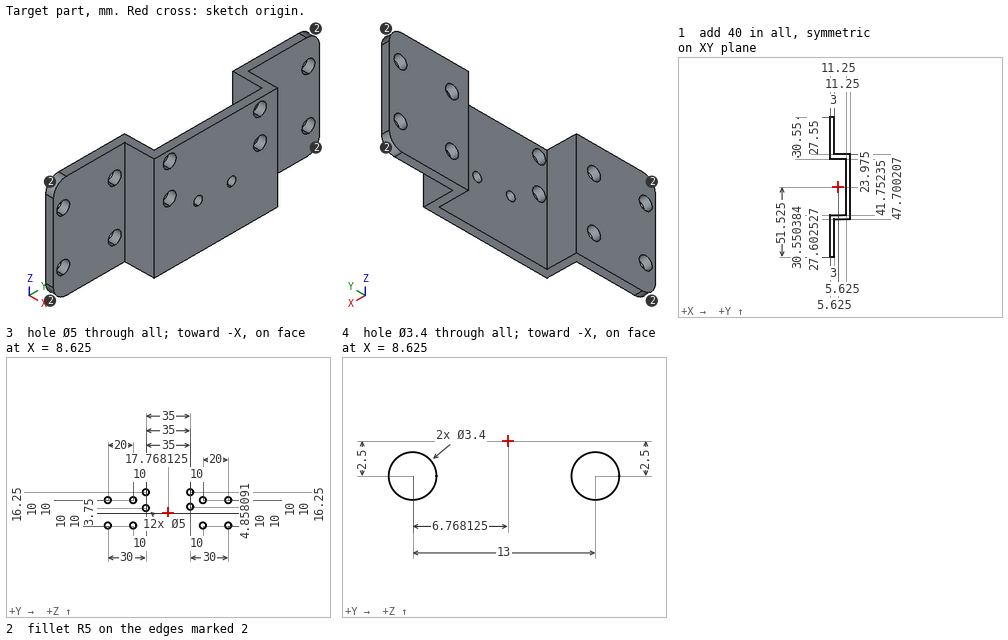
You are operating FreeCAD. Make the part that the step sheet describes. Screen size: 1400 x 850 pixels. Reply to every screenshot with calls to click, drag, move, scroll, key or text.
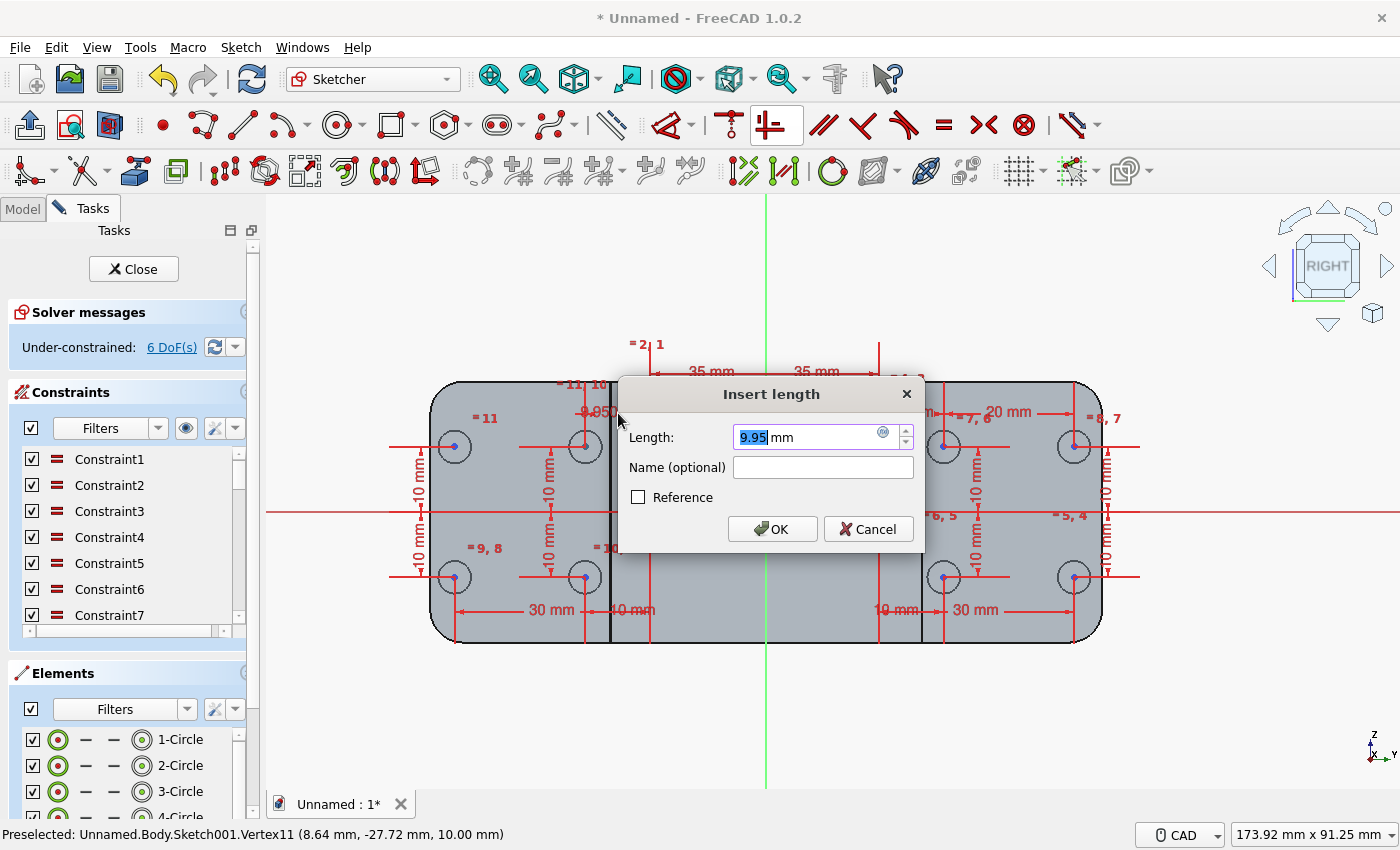
text(10)
key(Return)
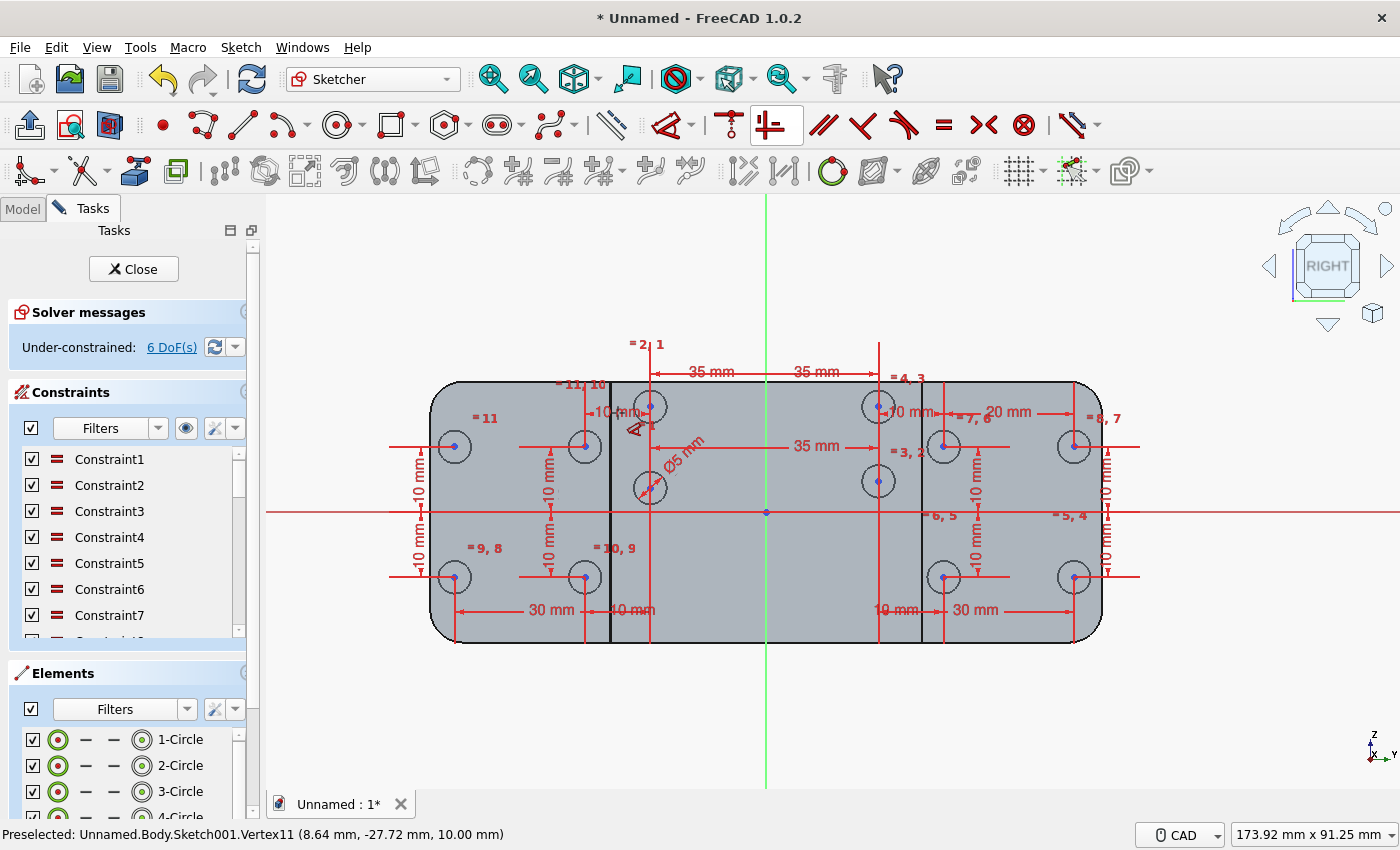
click(585, 447)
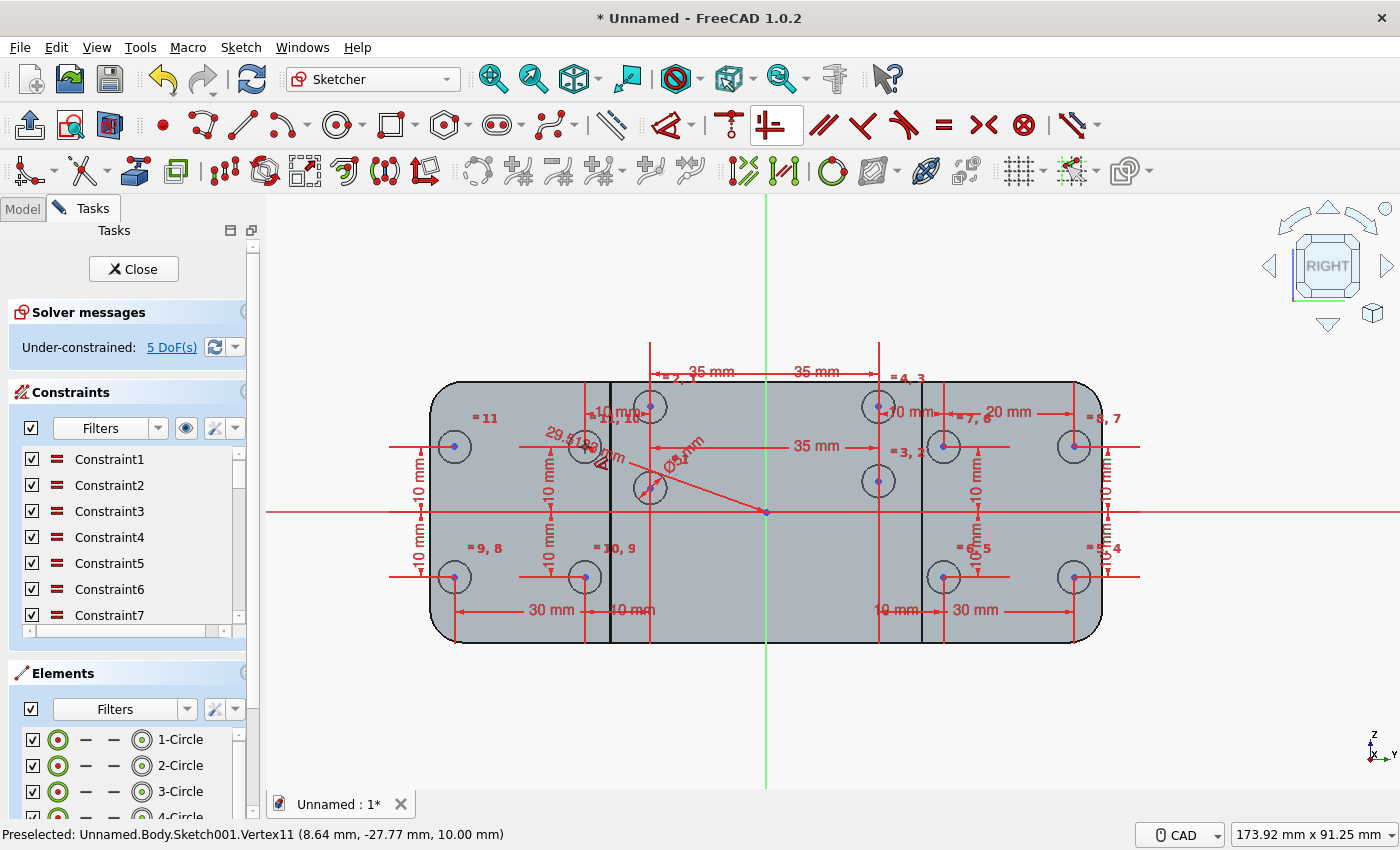
click(455, 447)
click(520, 413)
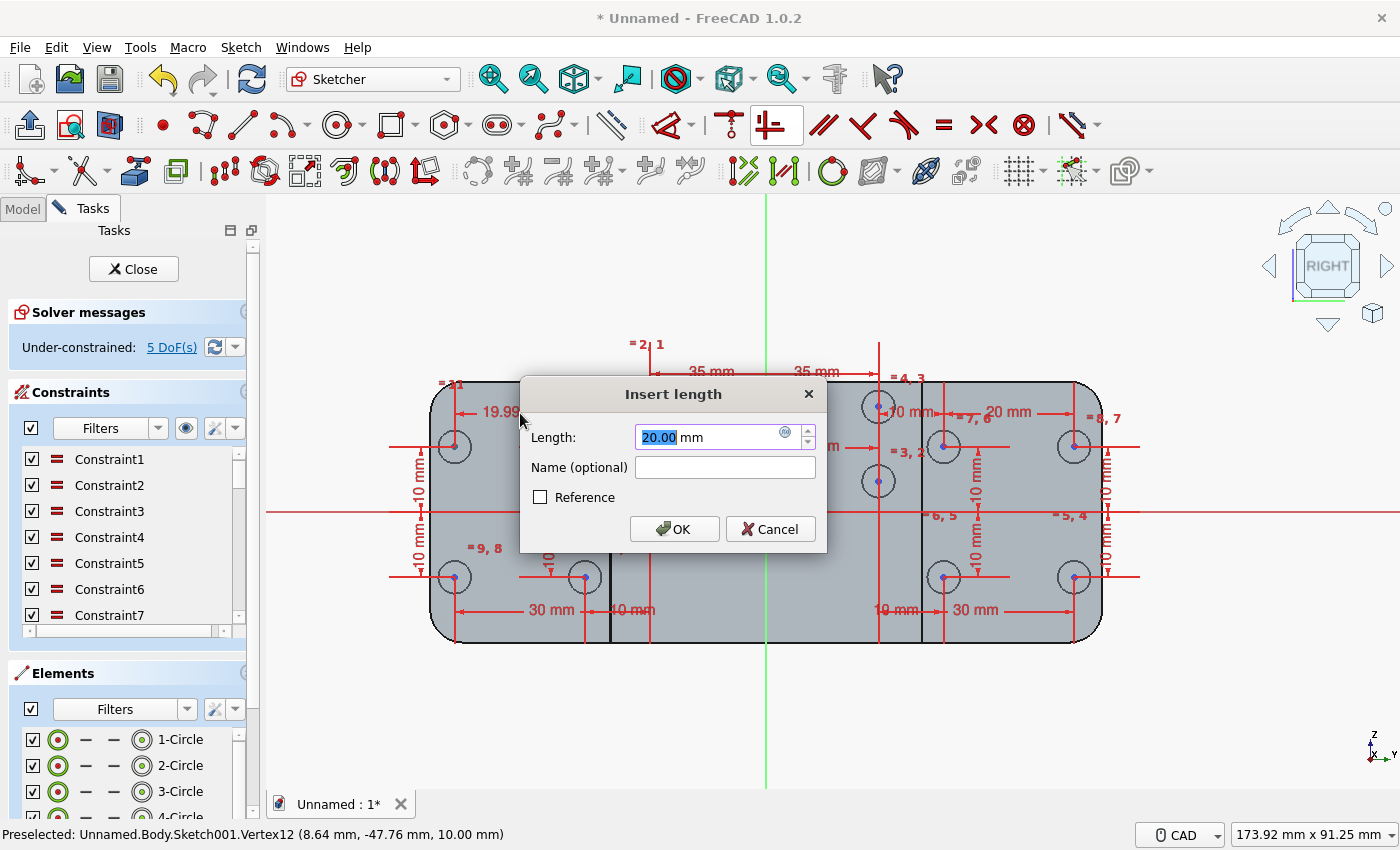
text(20)
key(Return)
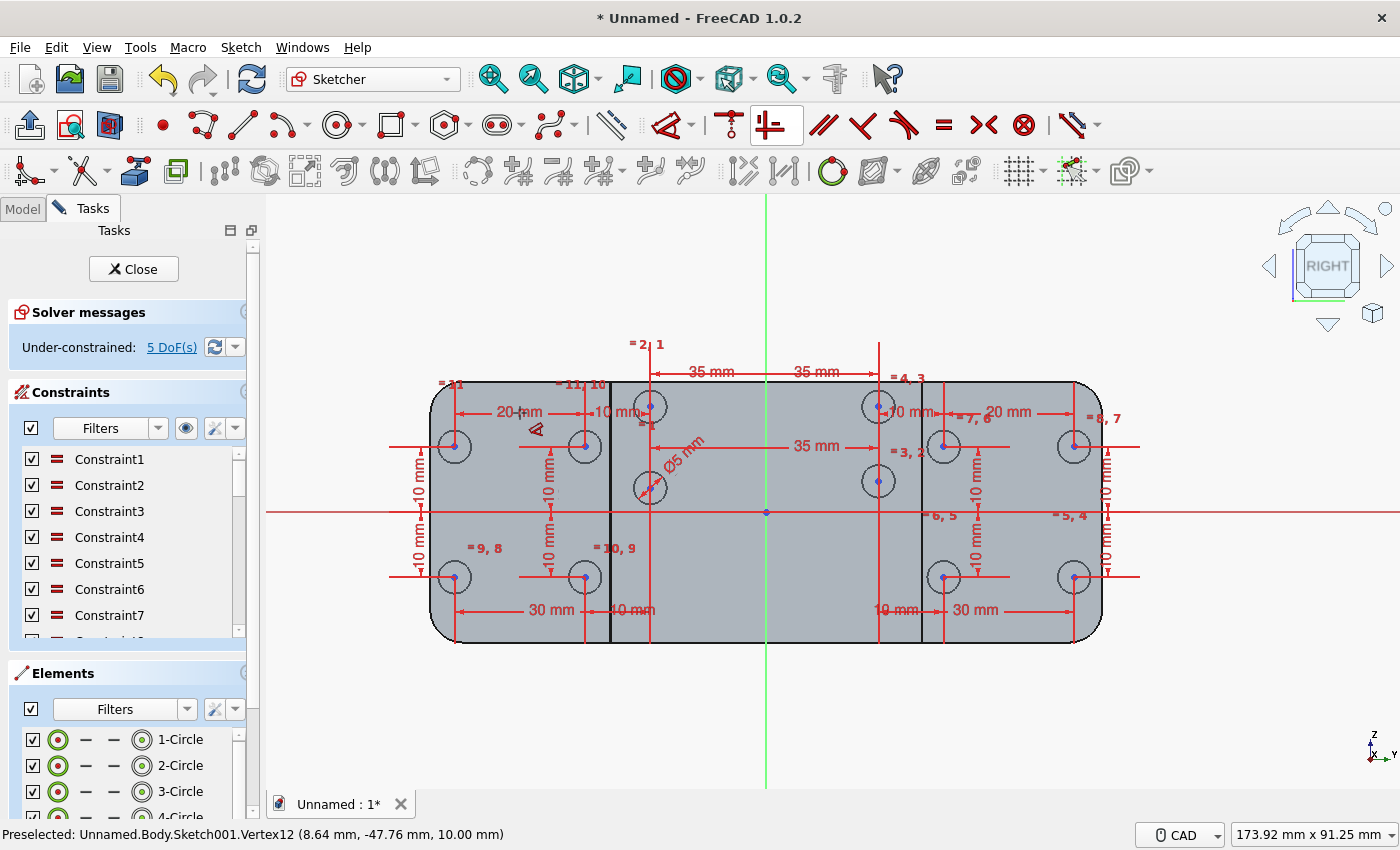
scroll(650, 488, up, 3)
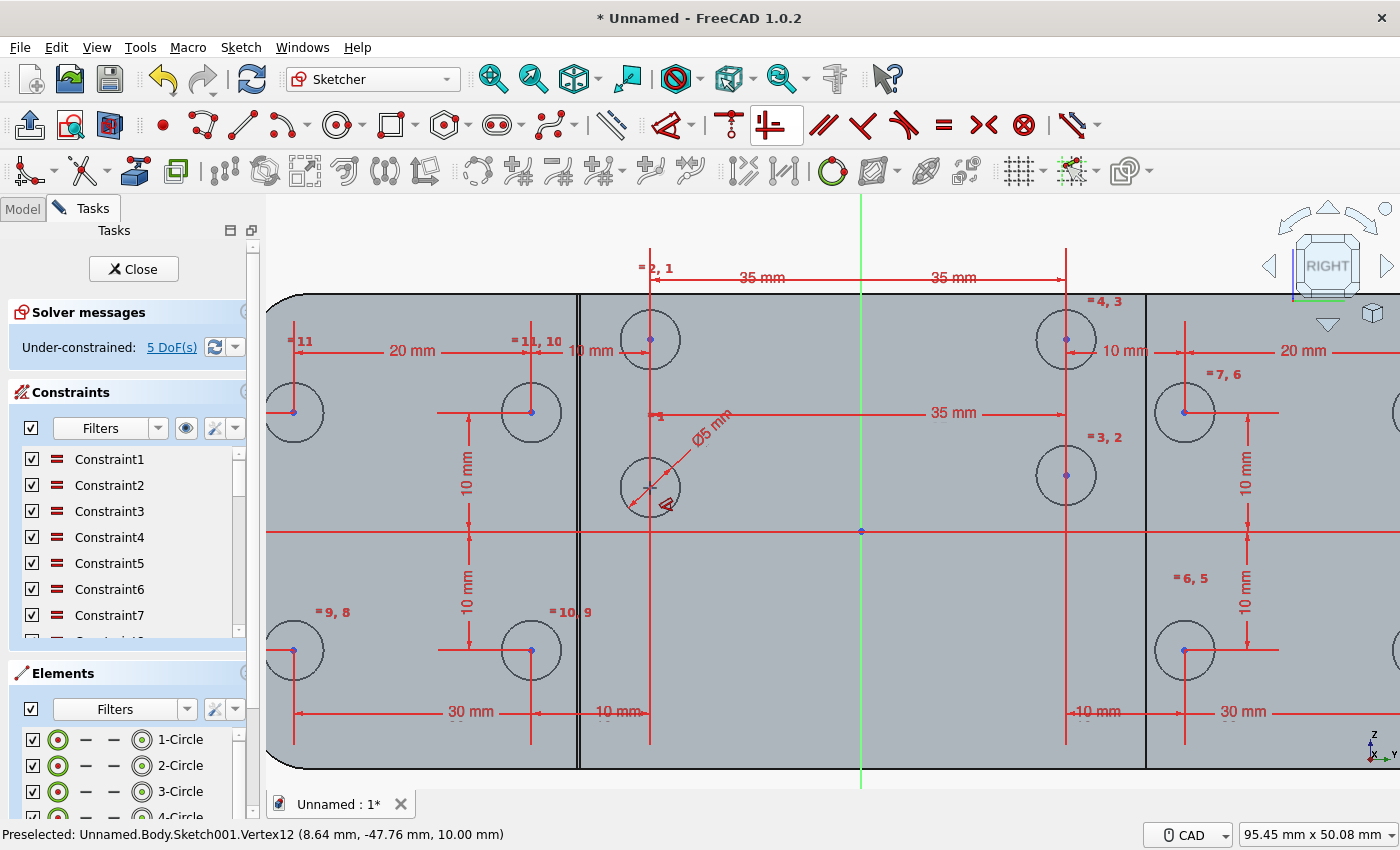
click(650, 488)
click(895, 510)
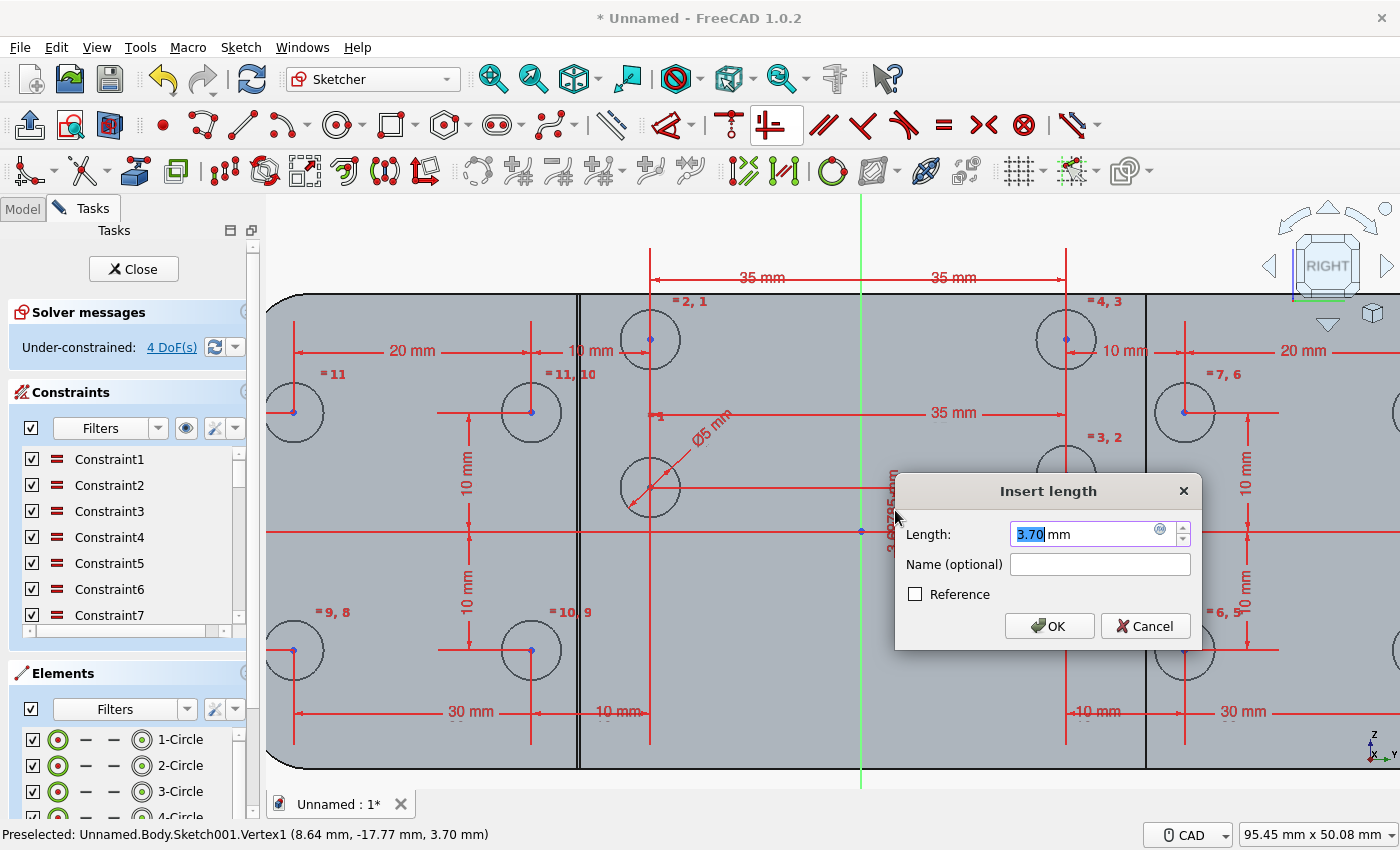
text(3.75)
key(Return)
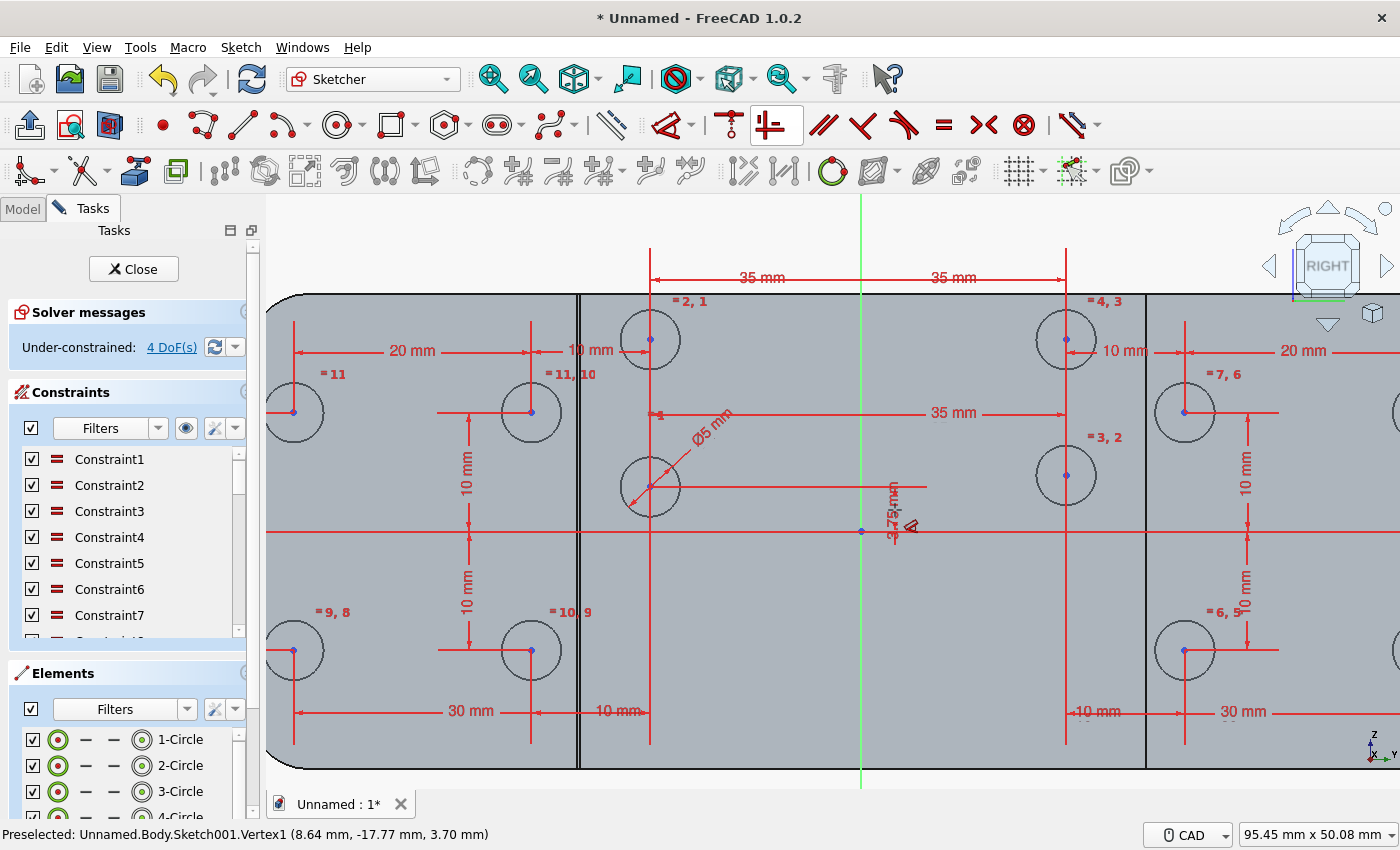
click(650, 340)
click(616, 436)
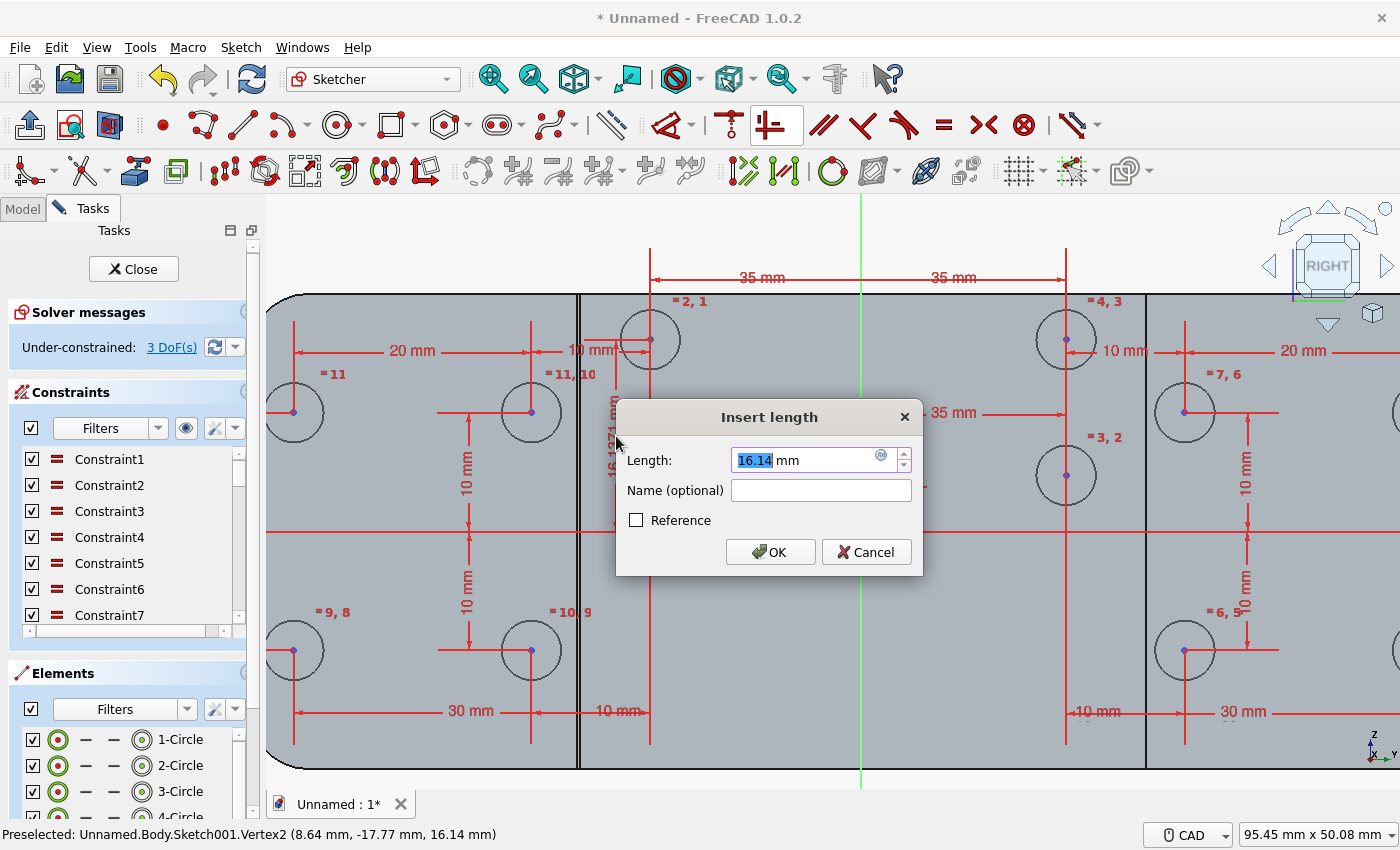
text(16.25)
key(Return)